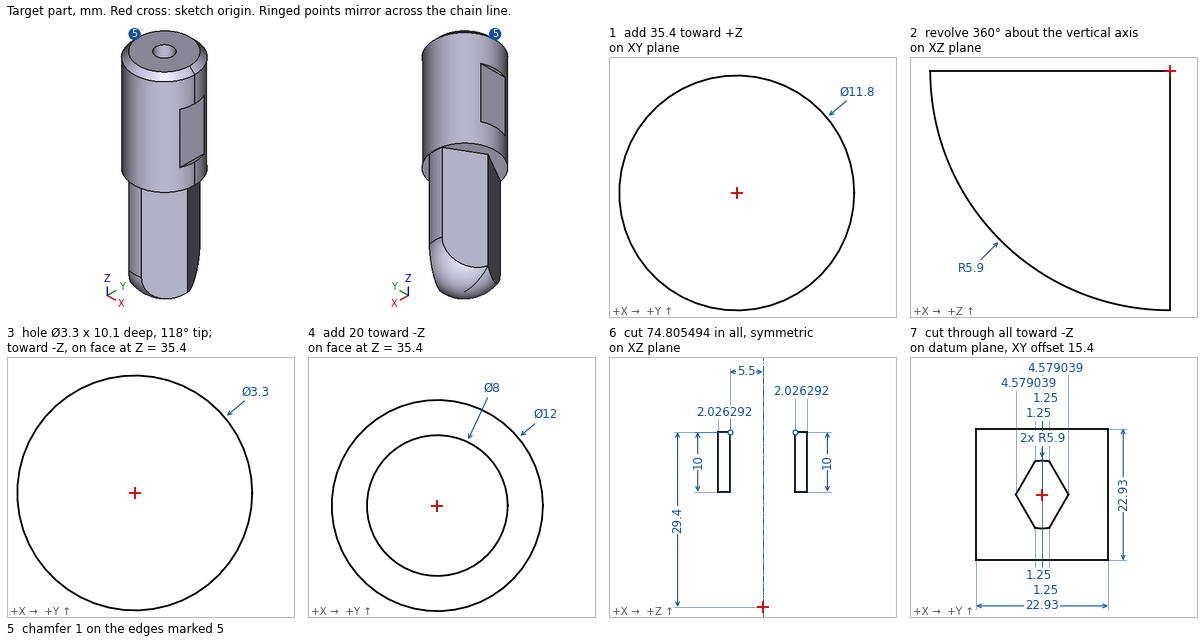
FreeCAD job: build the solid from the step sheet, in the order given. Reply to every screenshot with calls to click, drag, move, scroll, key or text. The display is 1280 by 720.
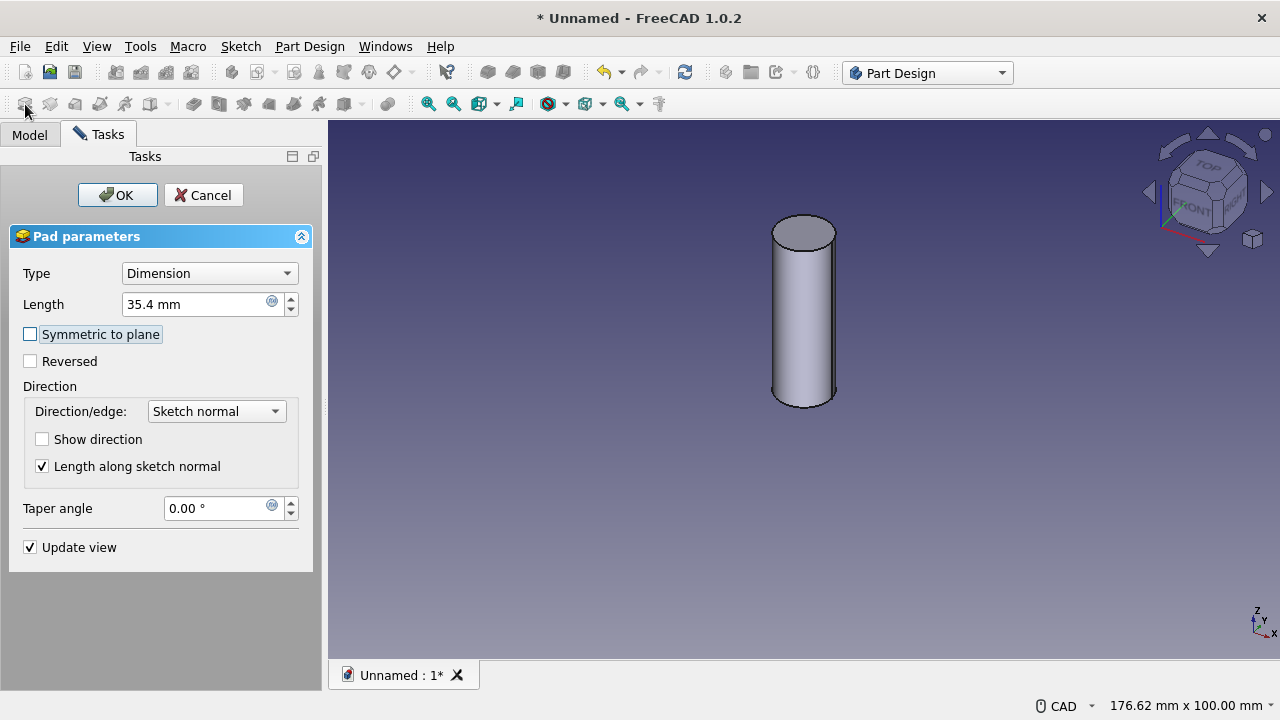
click(118, 195)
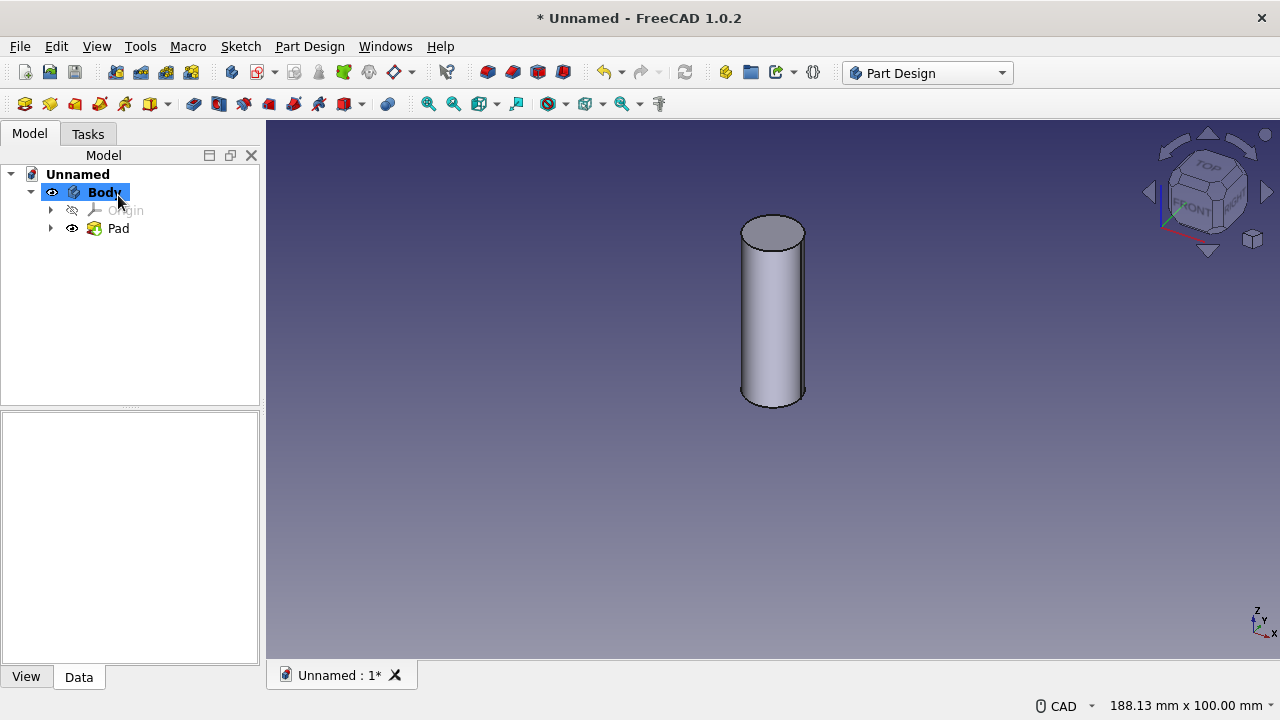
click(429, 104)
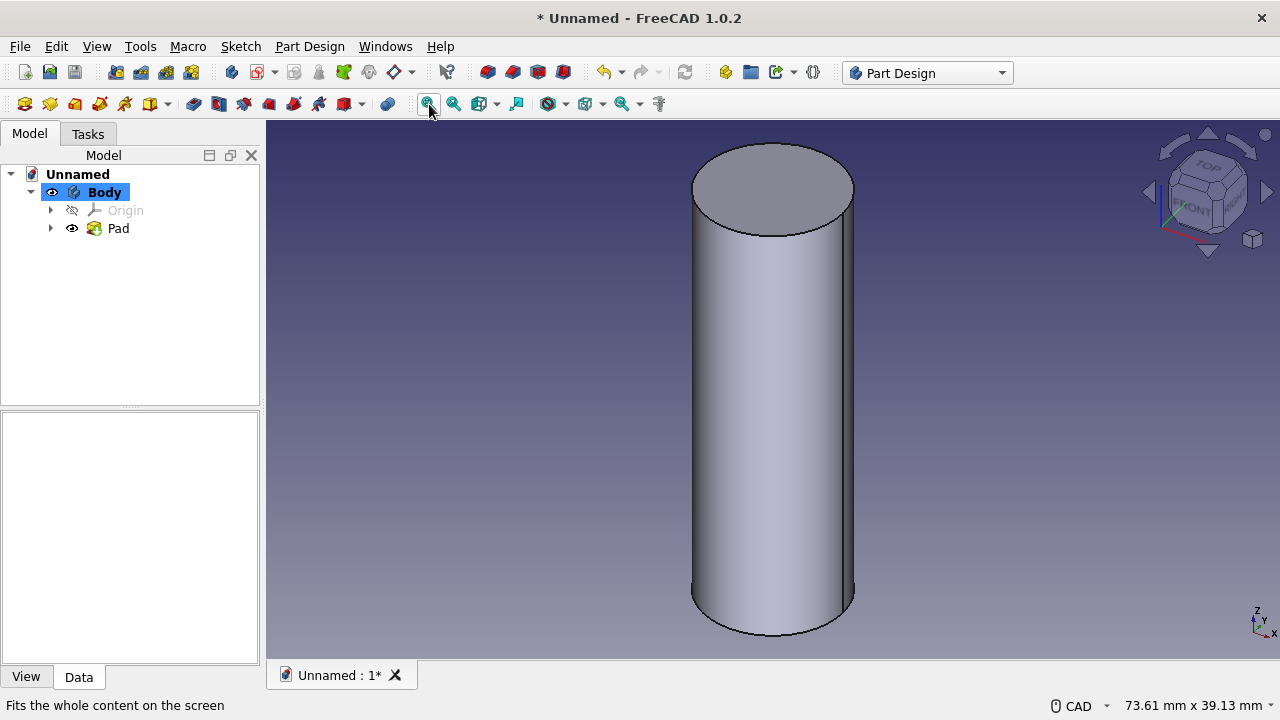
click(256, 72)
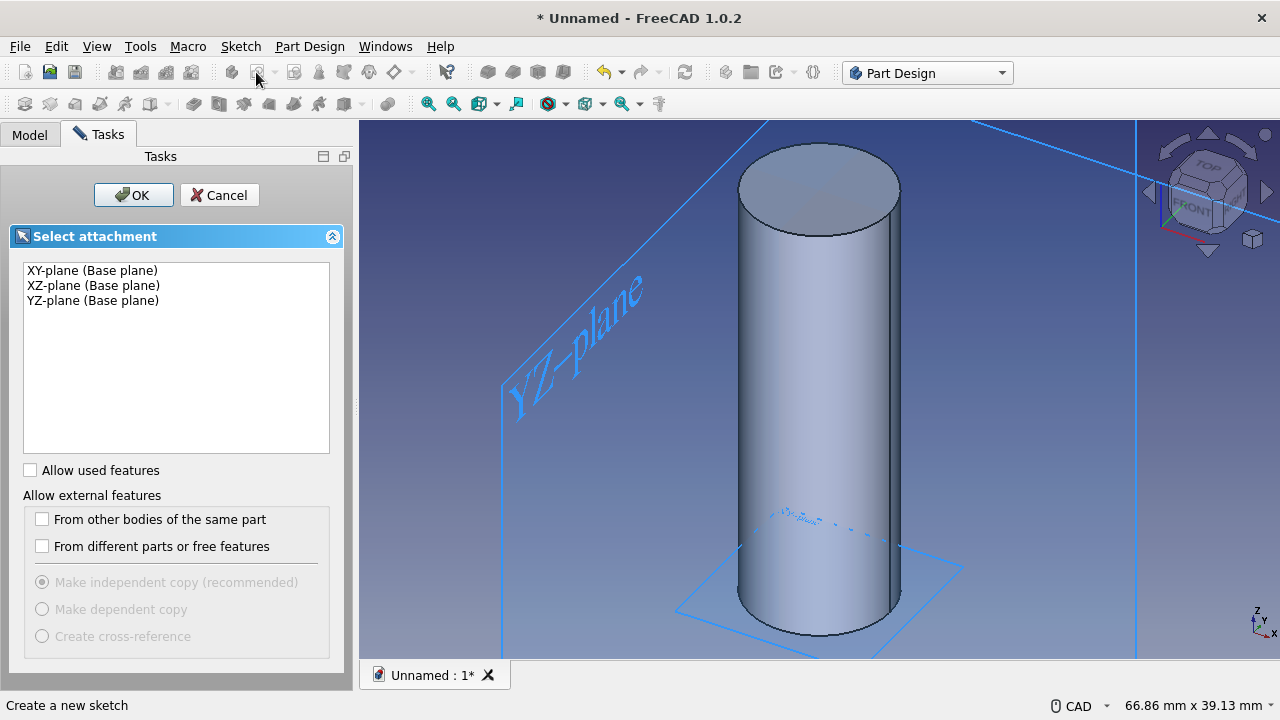
click(84, 286)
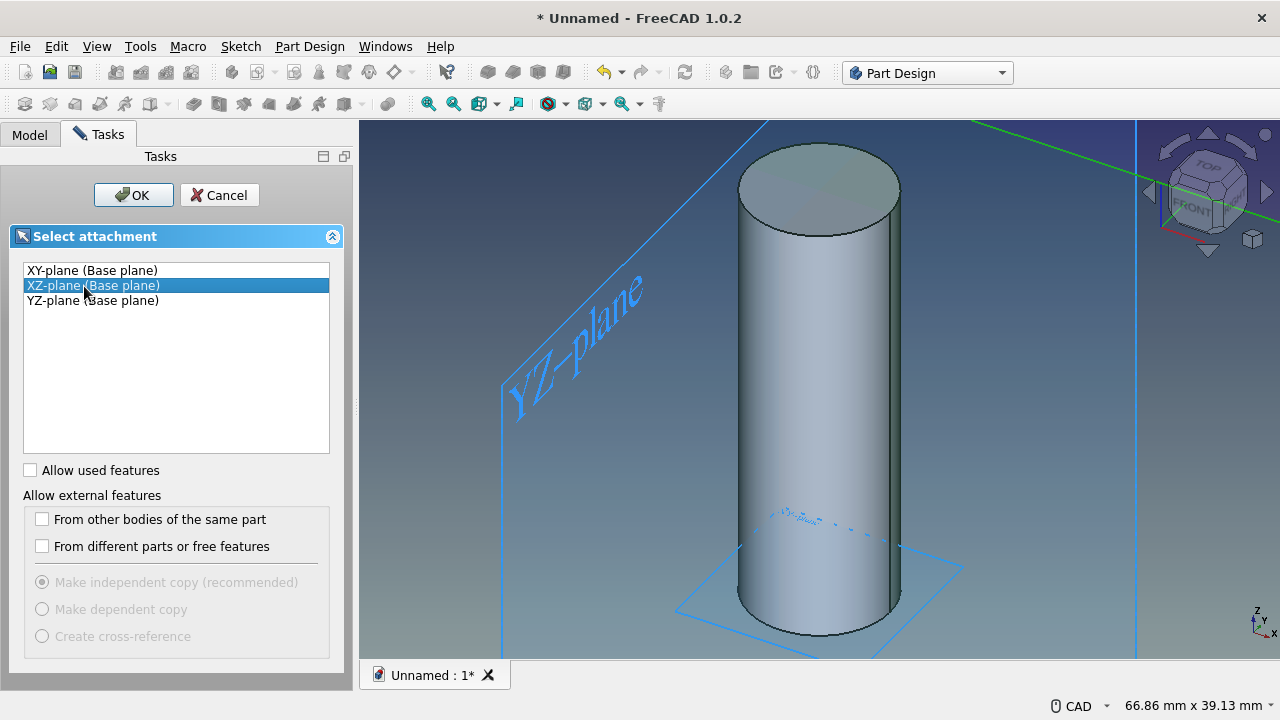
click(134, 195)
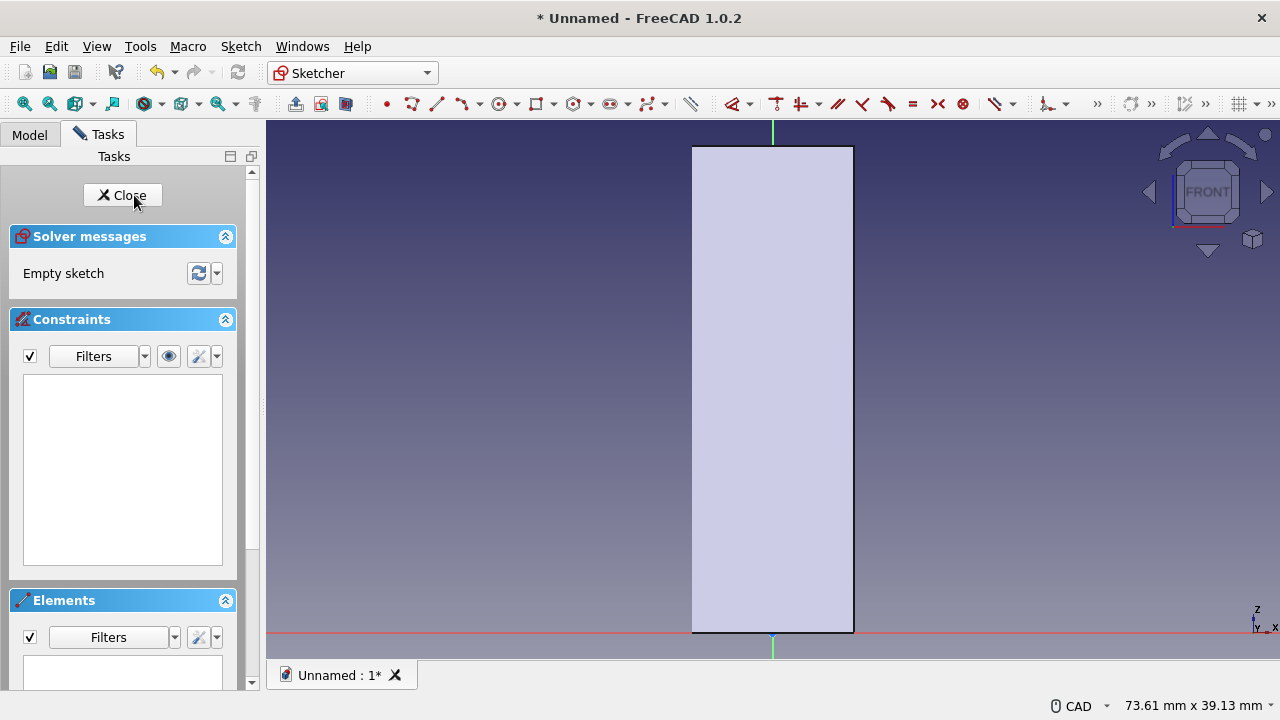
key(q)
key(s)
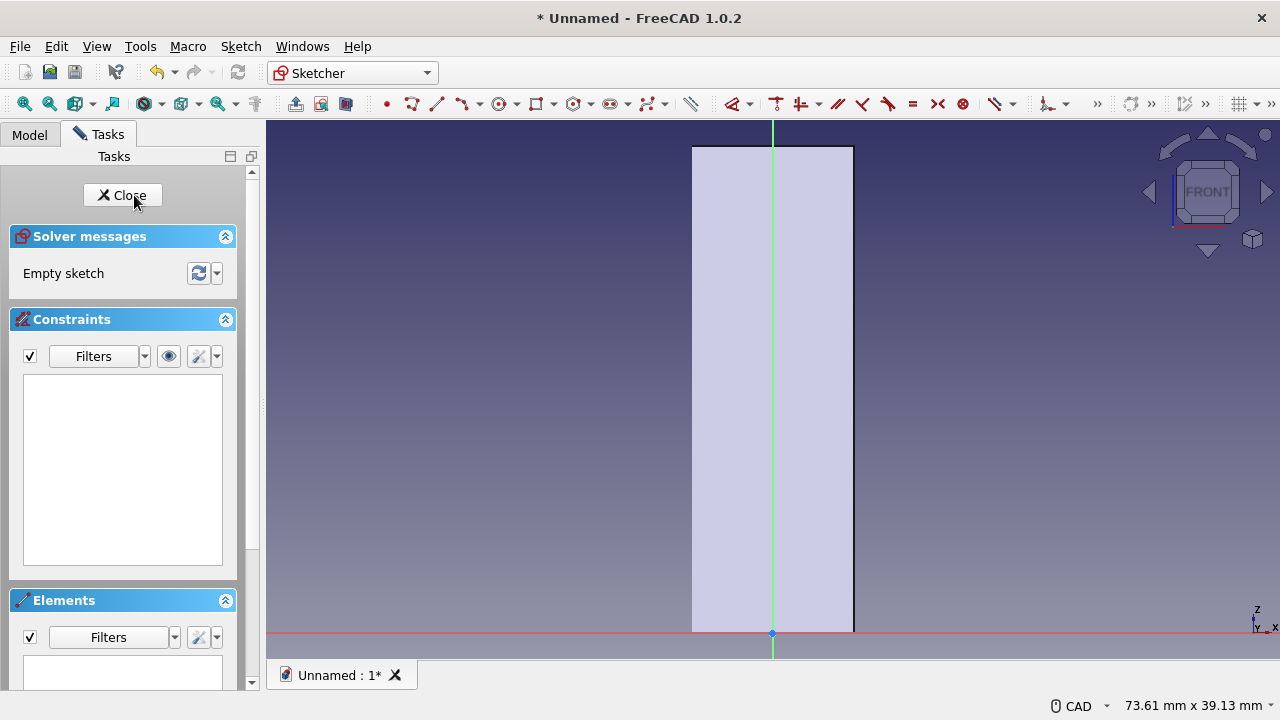
scroll(704, 390, down, 5)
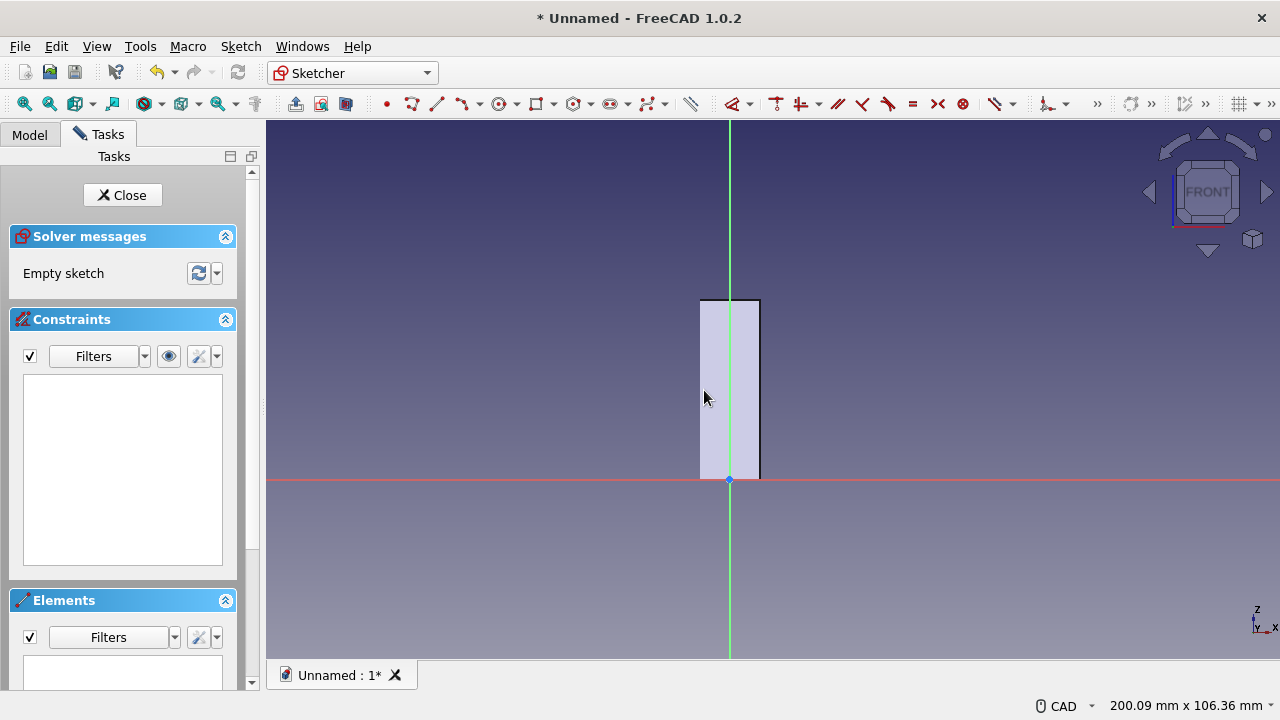
scroll(716, 505, up, 12)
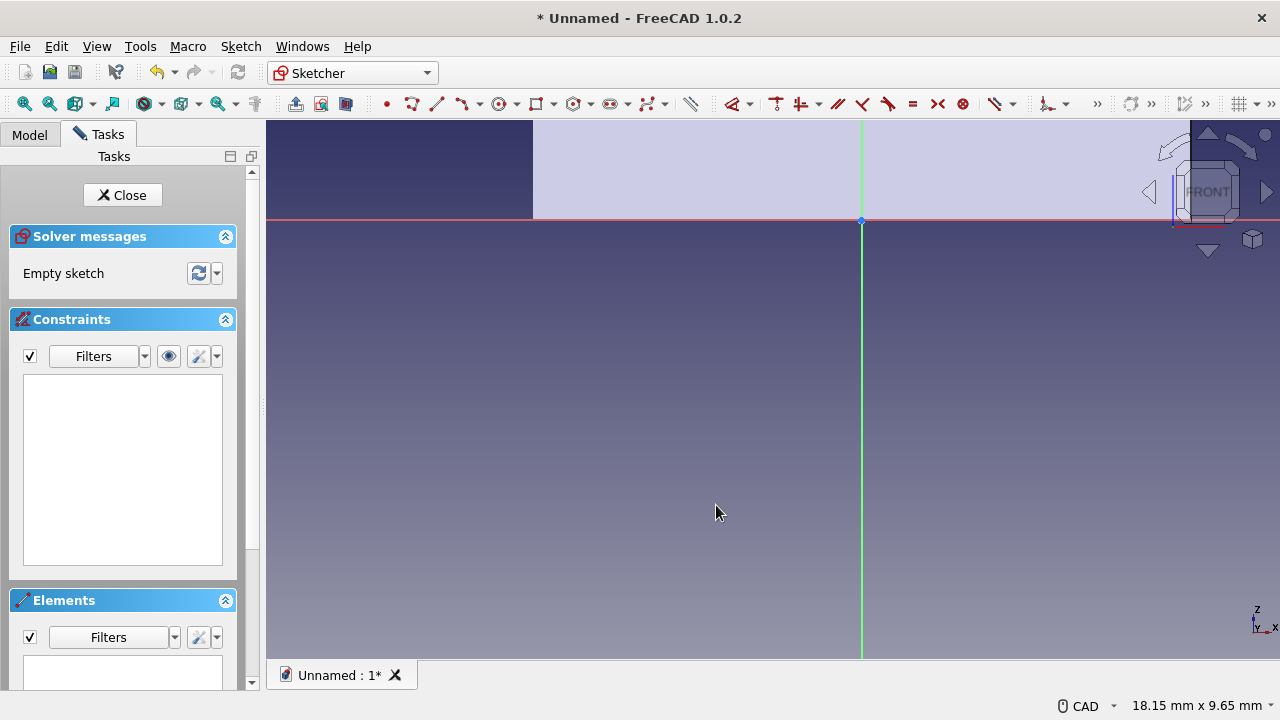
click(412, 104)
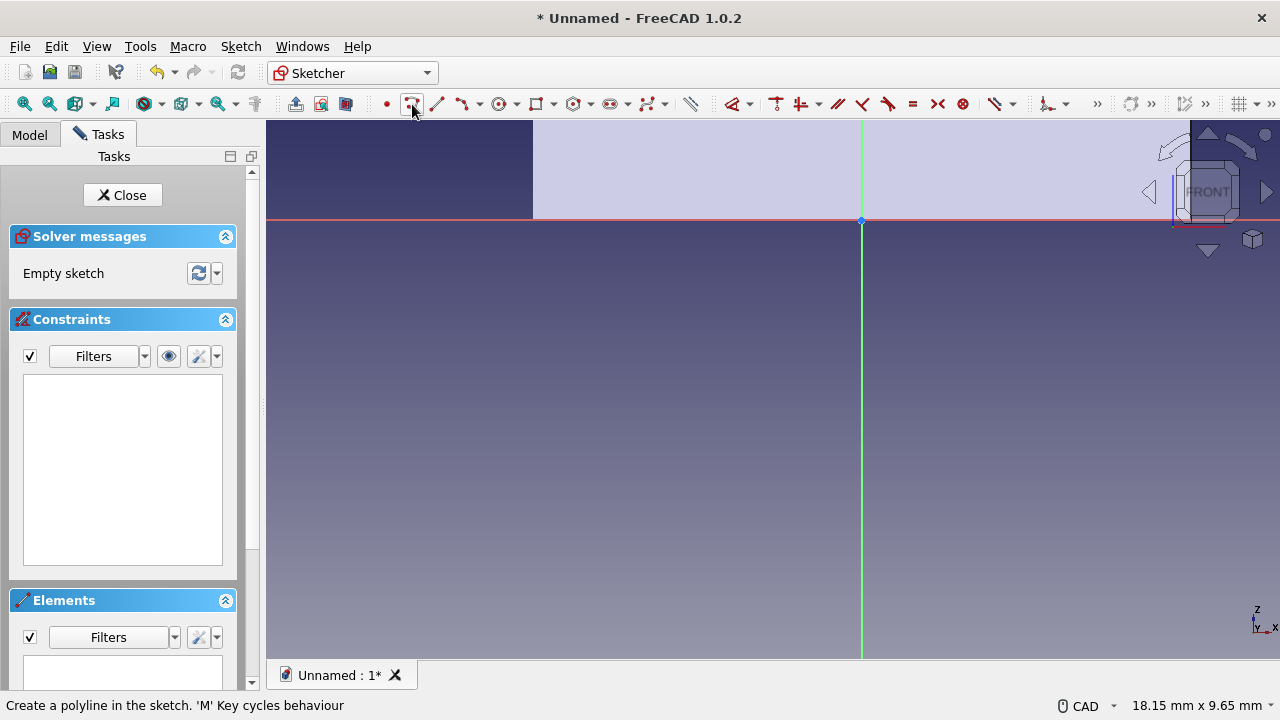
click(532, 220)
click(862, 220)
click(853, 550)
right_click(853, 550)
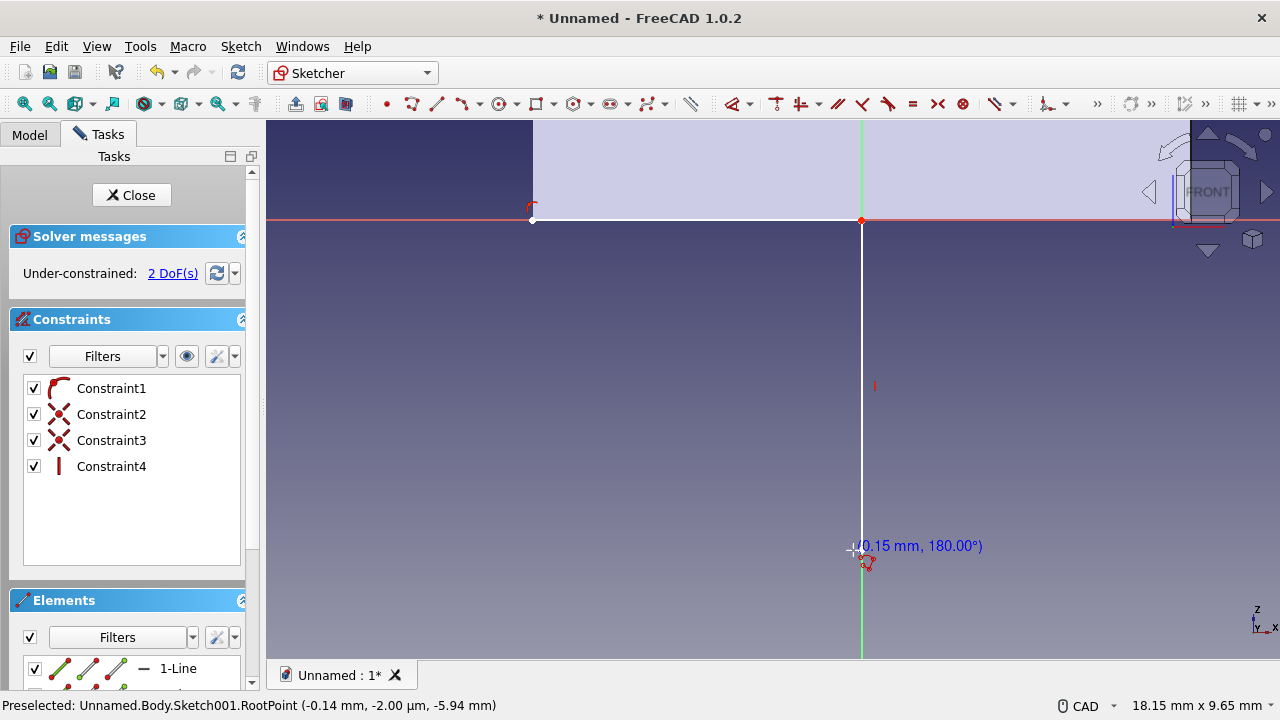
key(g)
key(3)
key(a)